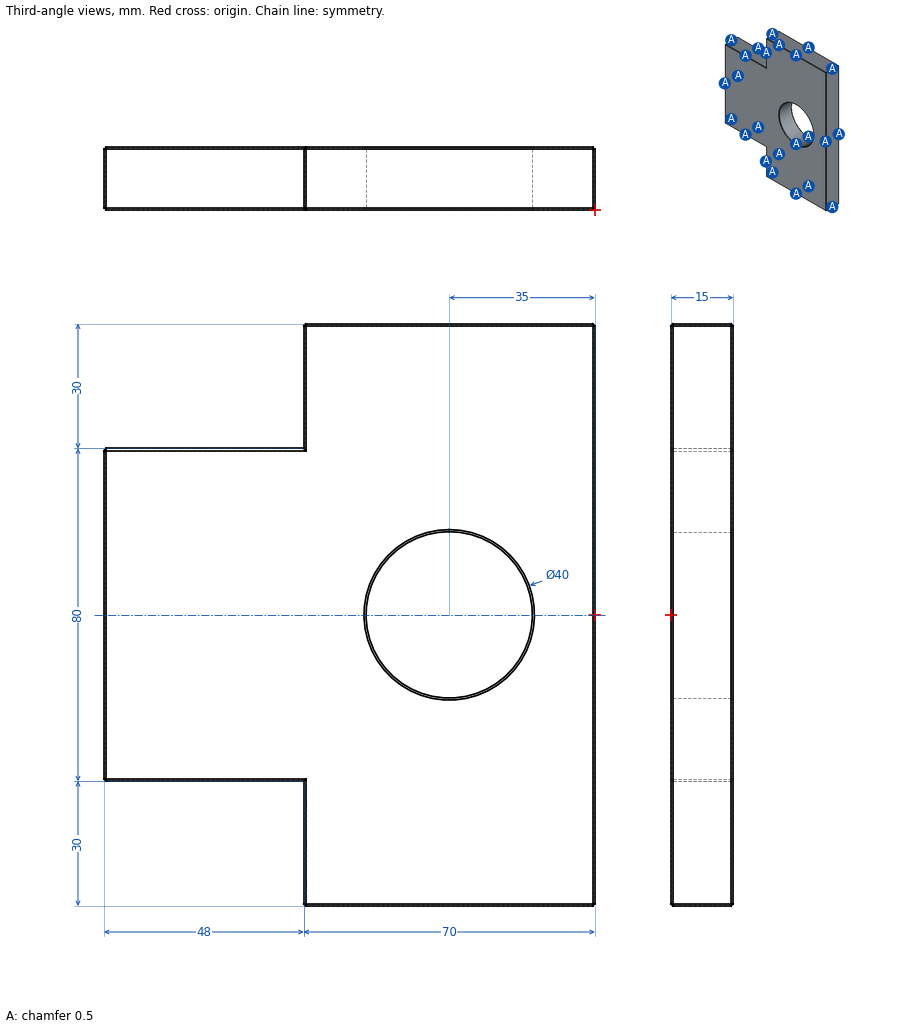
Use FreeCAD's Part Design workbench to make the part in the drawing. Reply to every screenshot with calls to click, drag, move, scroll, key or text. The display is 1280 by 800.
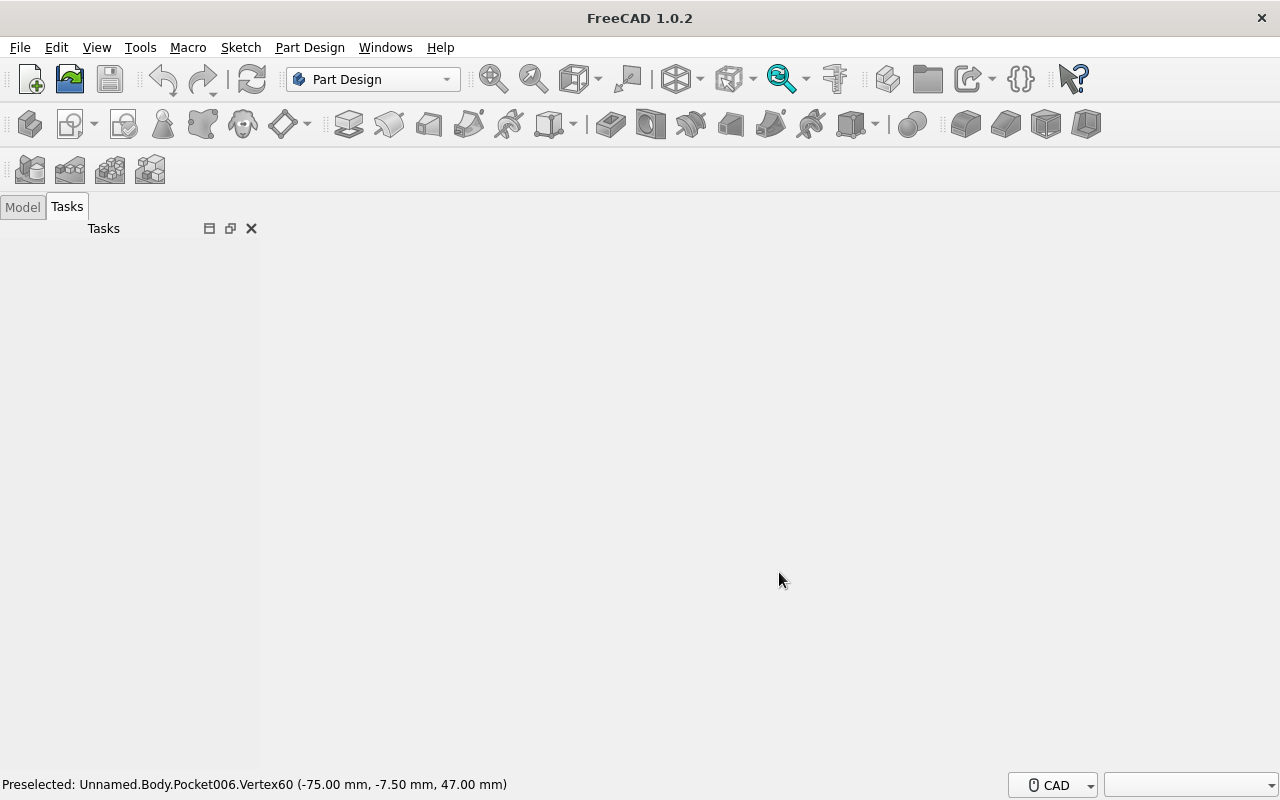
click(30, 80)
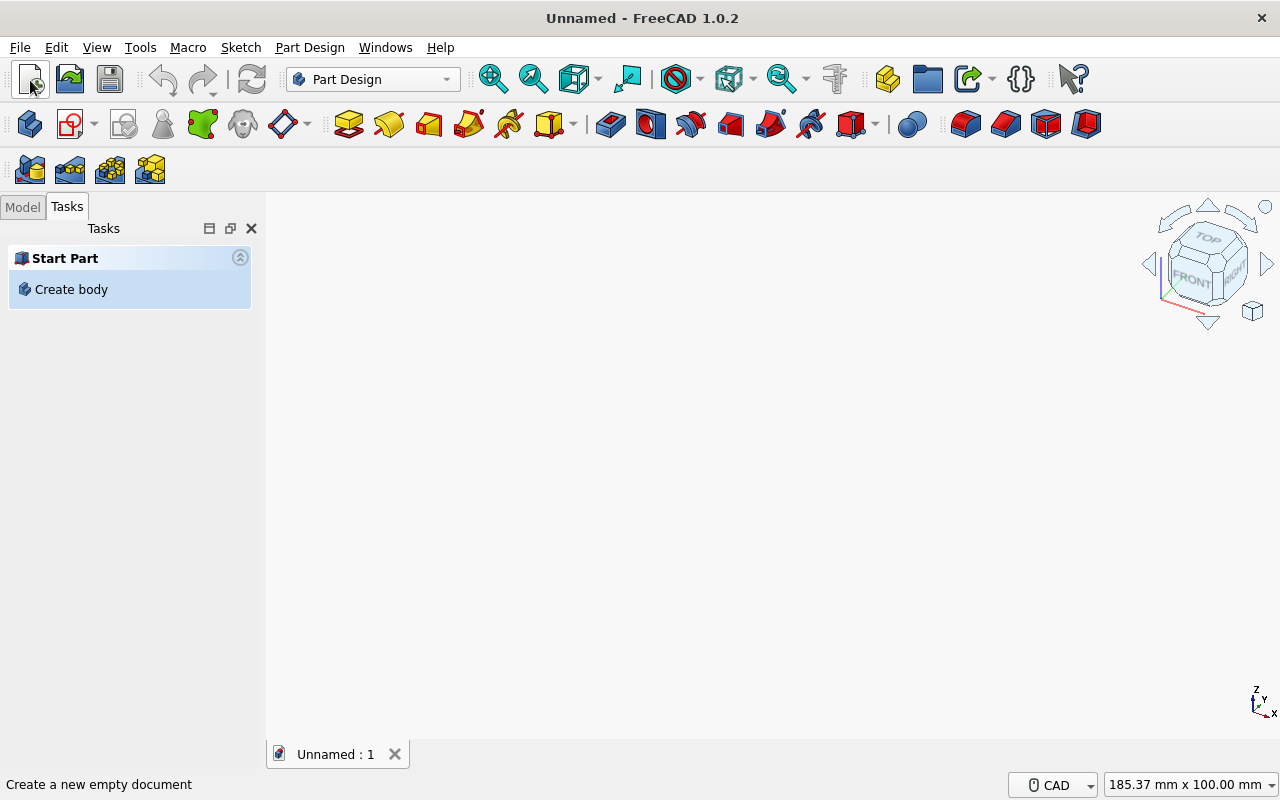
click(70, 124)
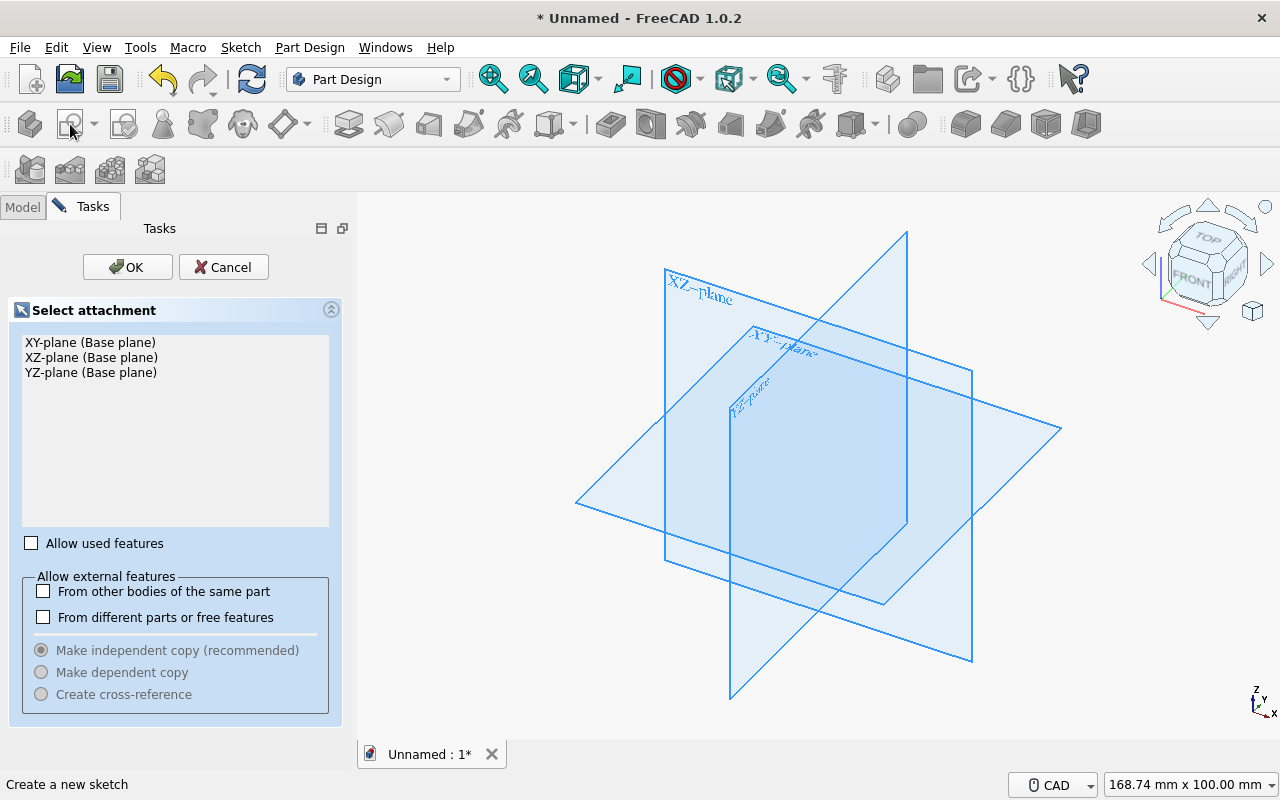
click(82, 358)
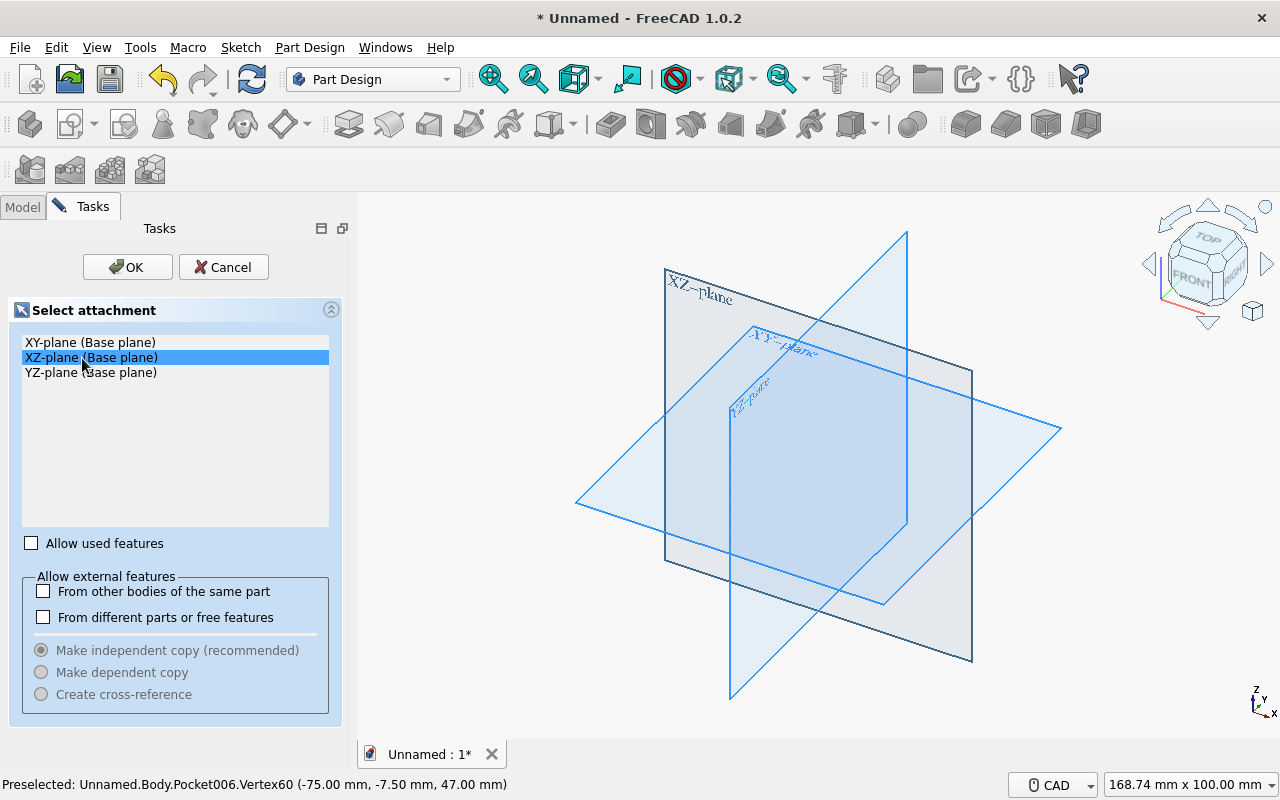
click(128, 267)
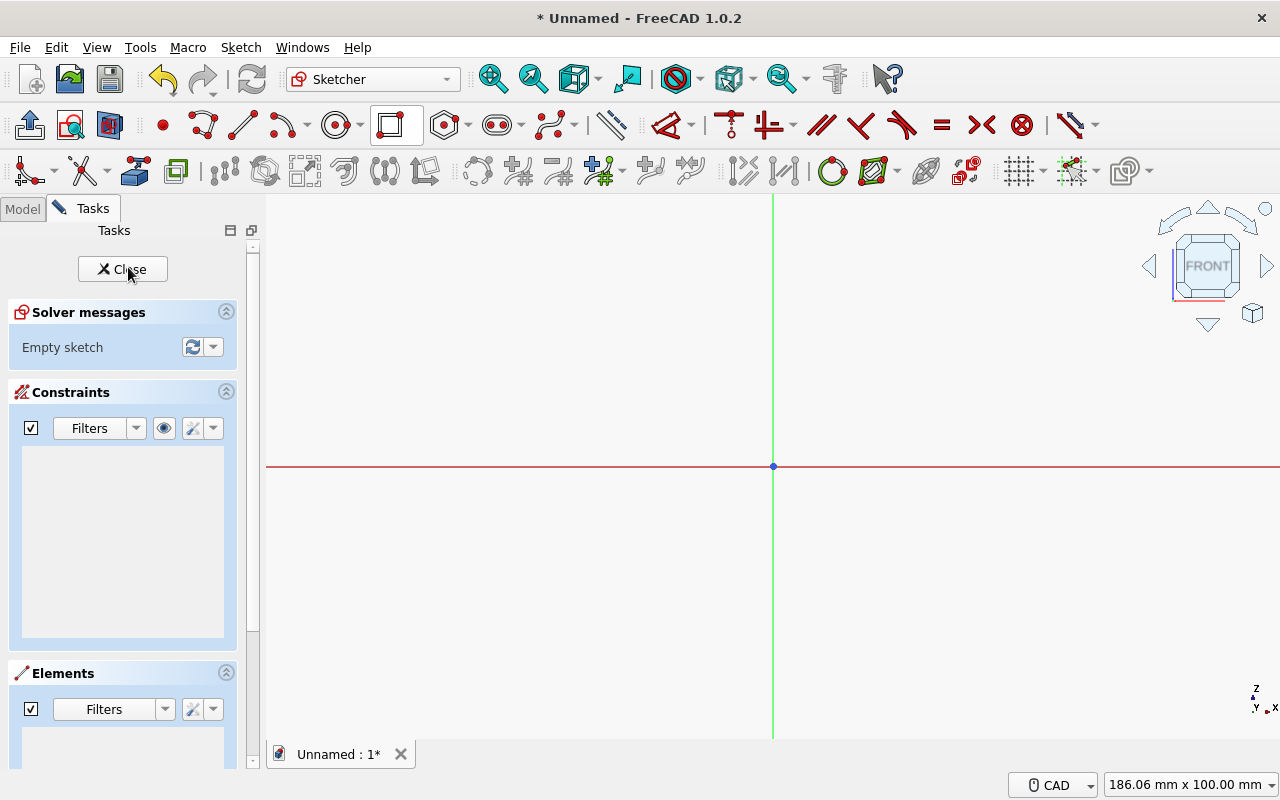
scroll(911, 466, down, 4)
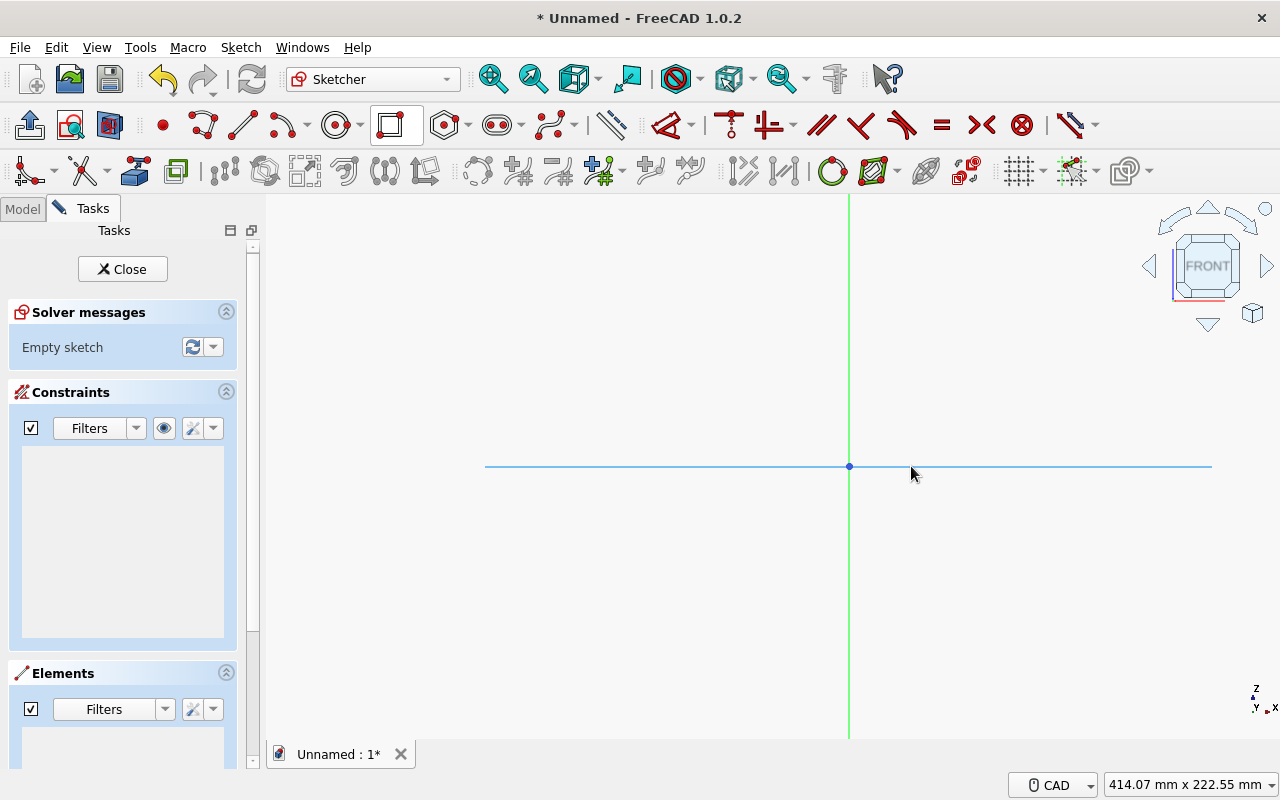
key(g)
key(m)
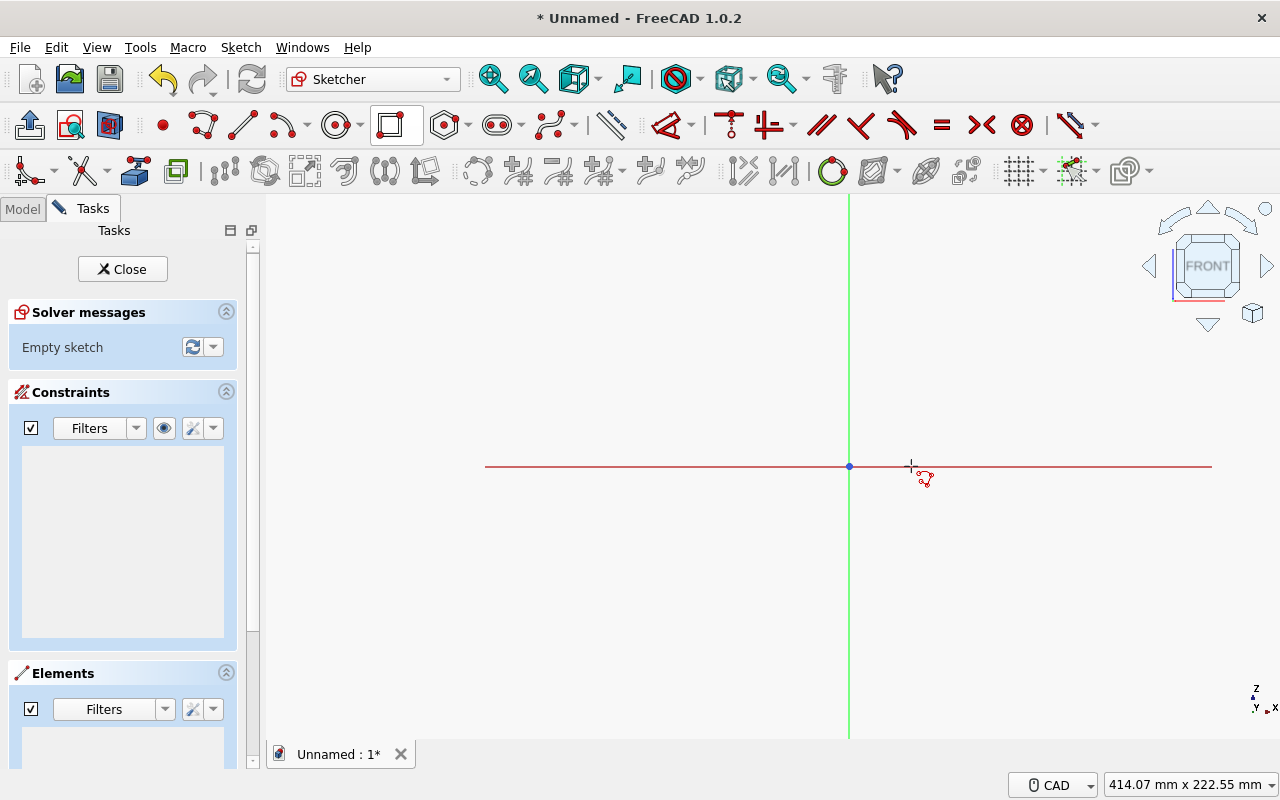
click(849, 295)
click(840, 638)
click(678, 638)
click(678, 564)
click(560, 564)
click(560, 369)
click(678, 369)
click(678, 295)
click(849, 296)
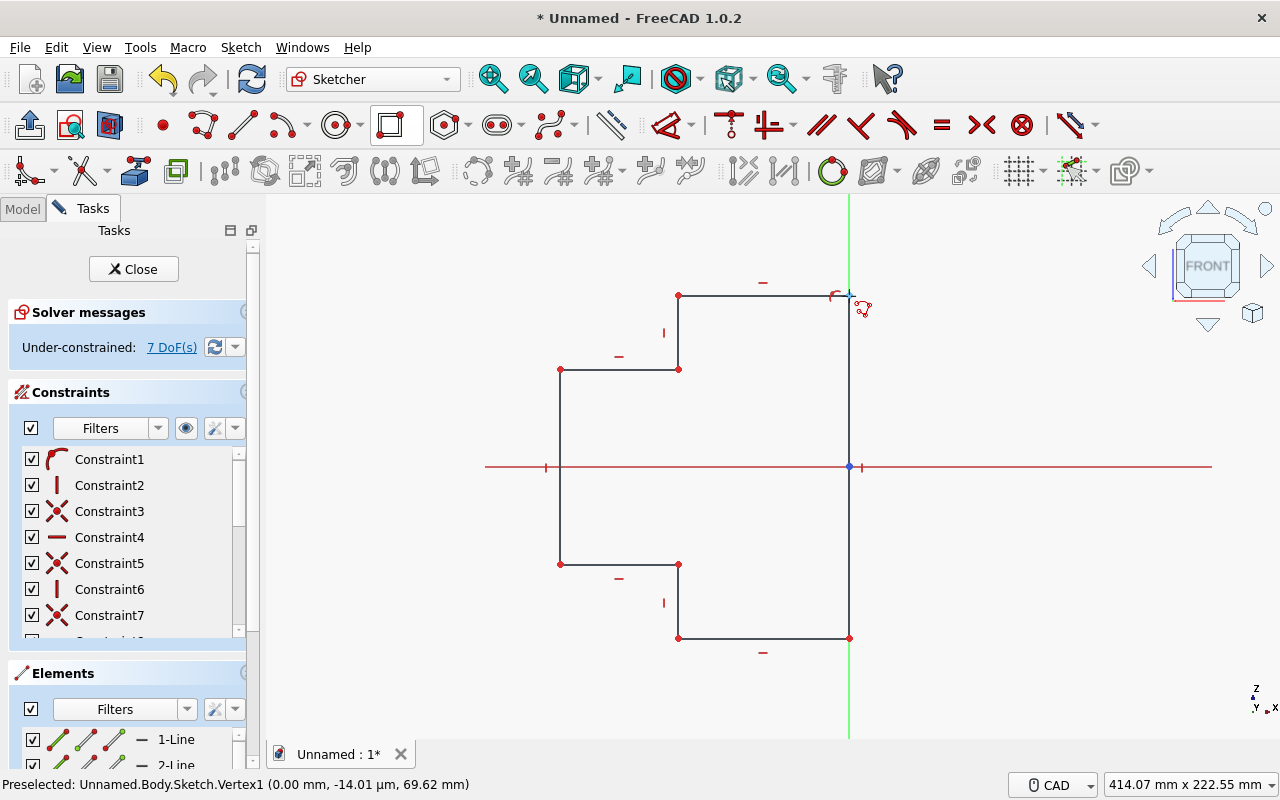
key(g)
key(c)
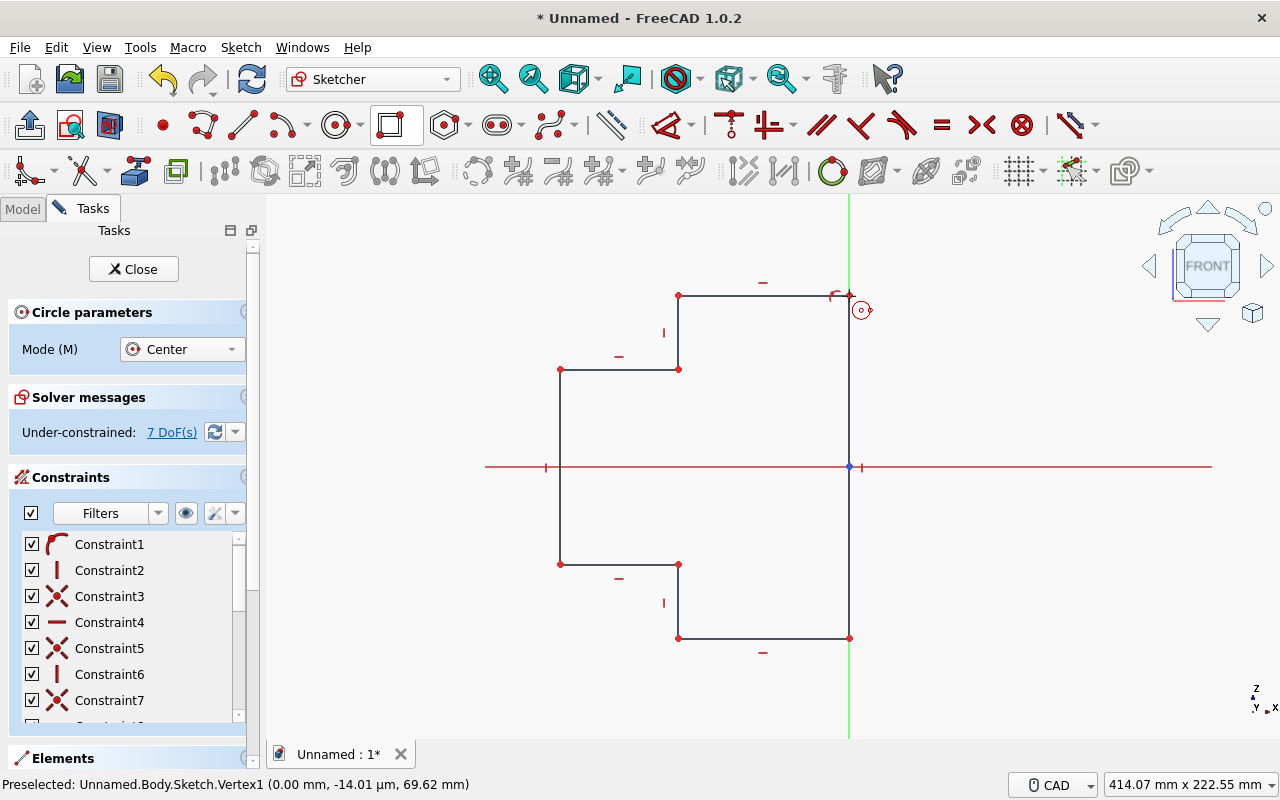
click(764, 466)
click(798, 432)
key(Escape)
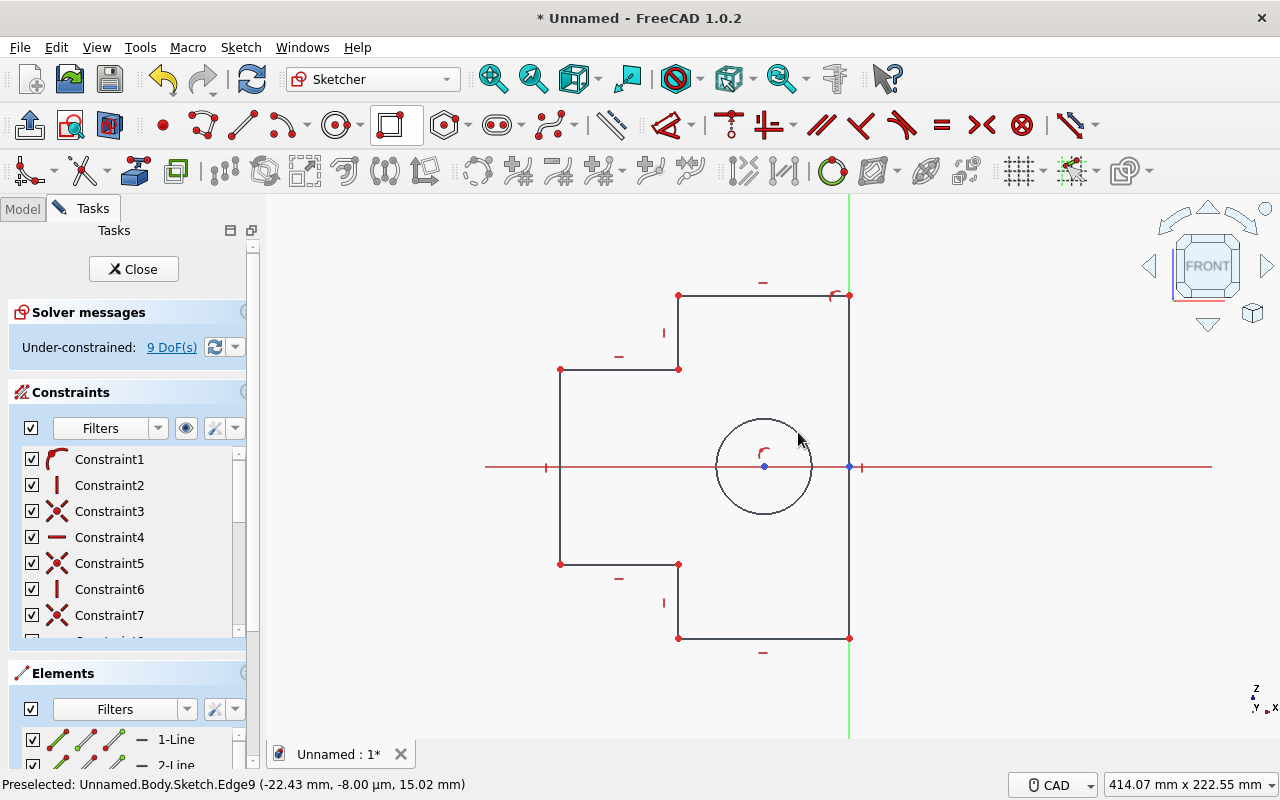
click(678, 565)